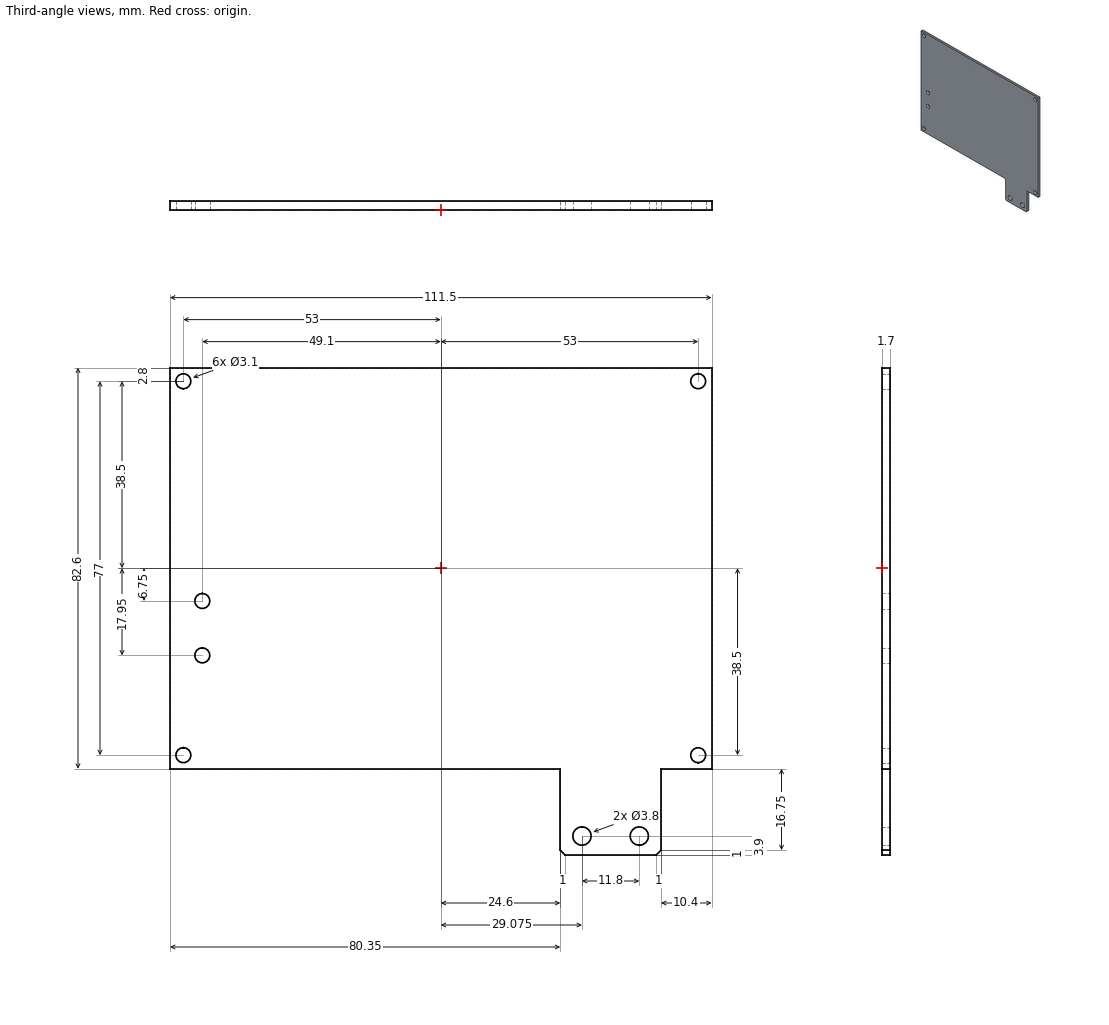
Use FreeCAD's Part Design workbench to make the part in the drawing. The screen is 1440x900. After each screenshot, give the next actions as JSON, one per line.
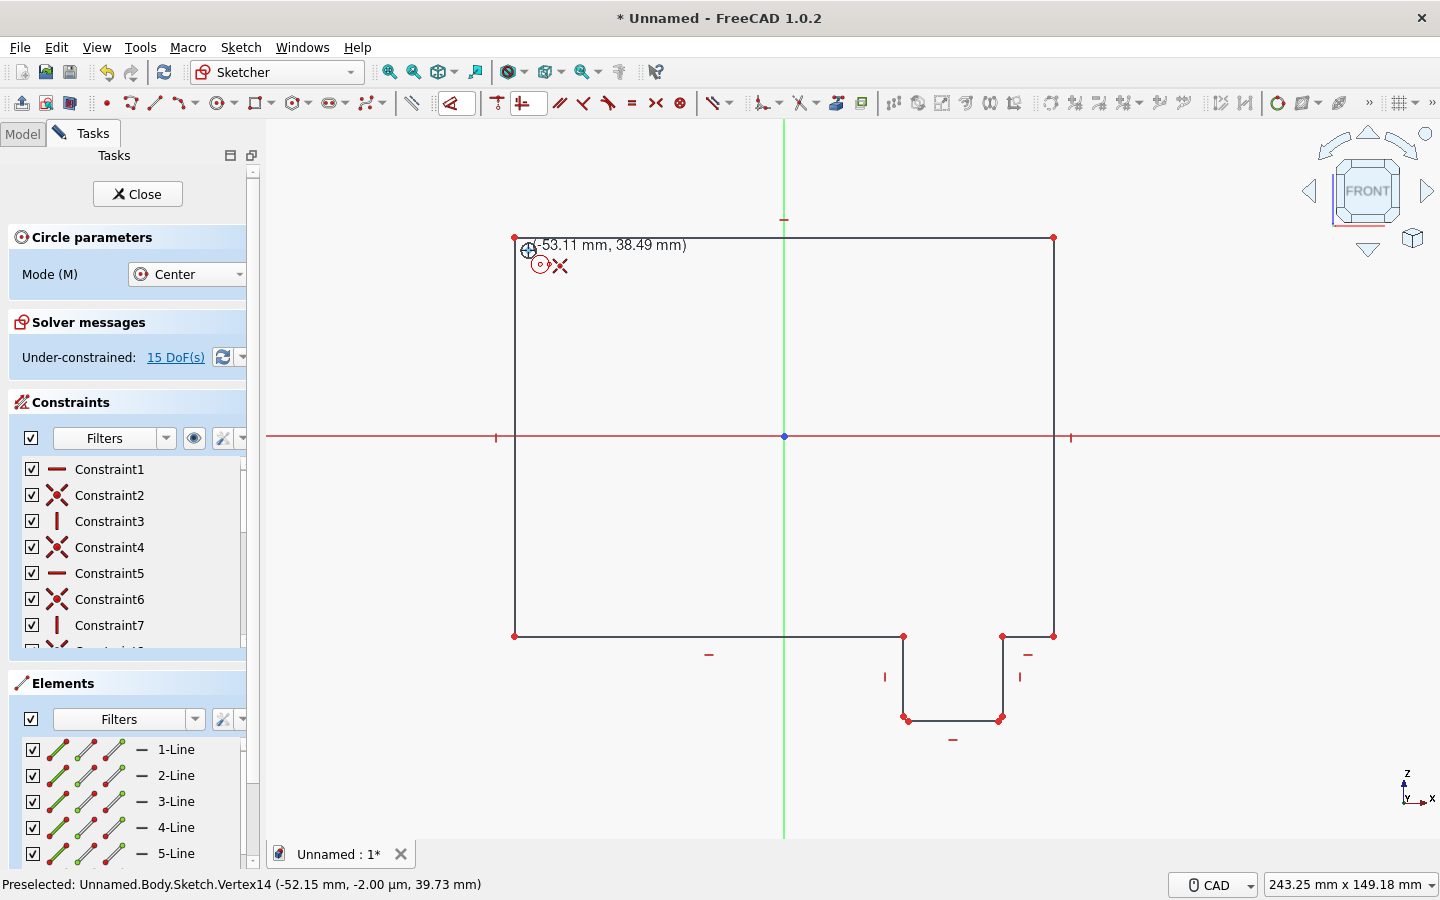
{"action": "scroll", "coordinate": [547, 469], "scroll_direction": "up", "scroll_amount": 6}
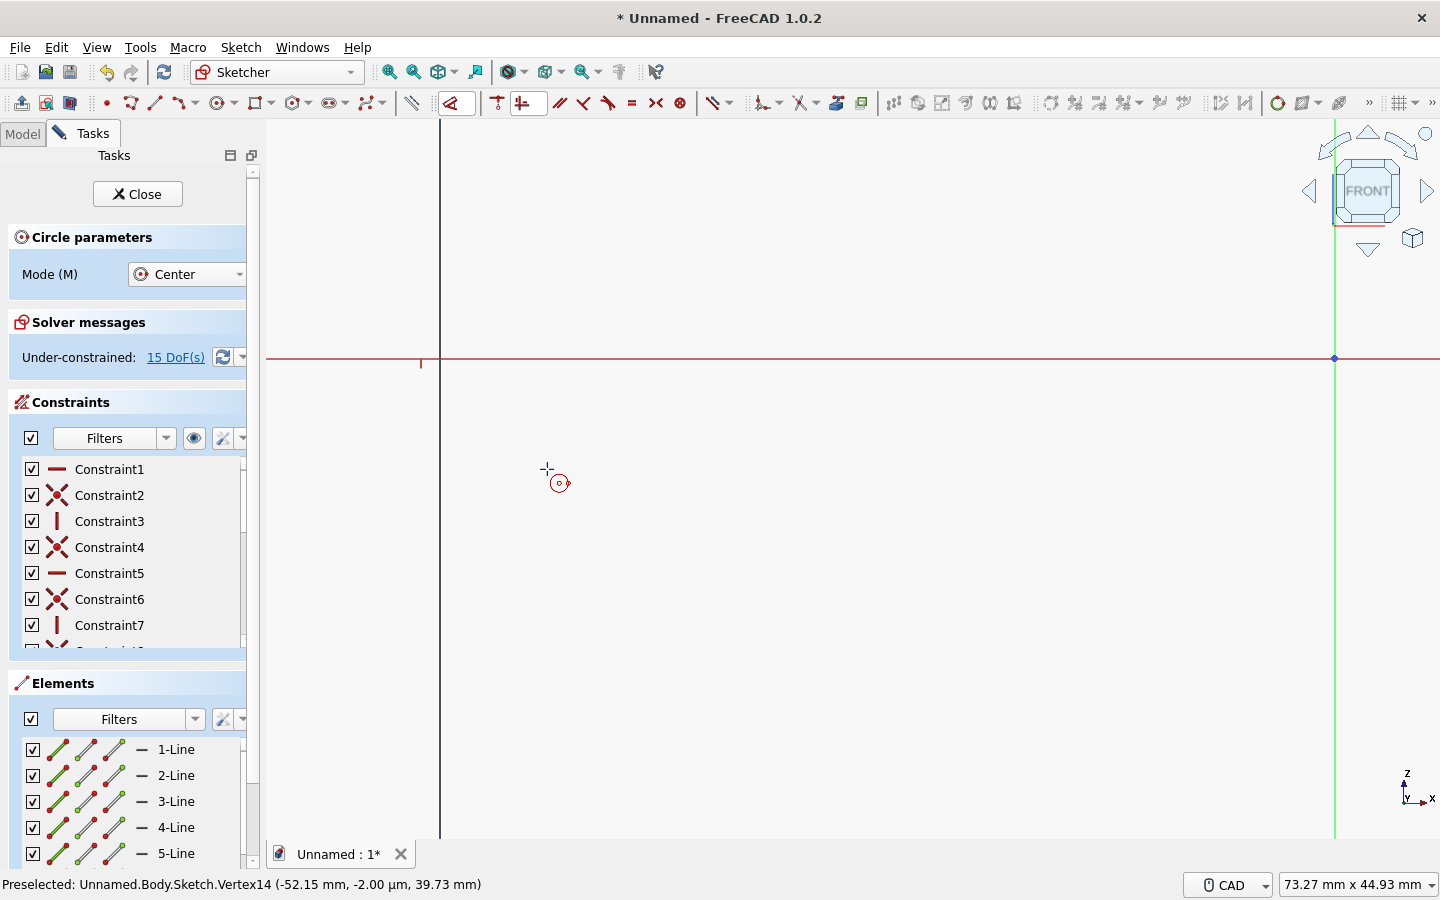
{"action": "left_click", "coordinate": [548, 467]}
{"action": "left_click", "coordinate": [566, 450]}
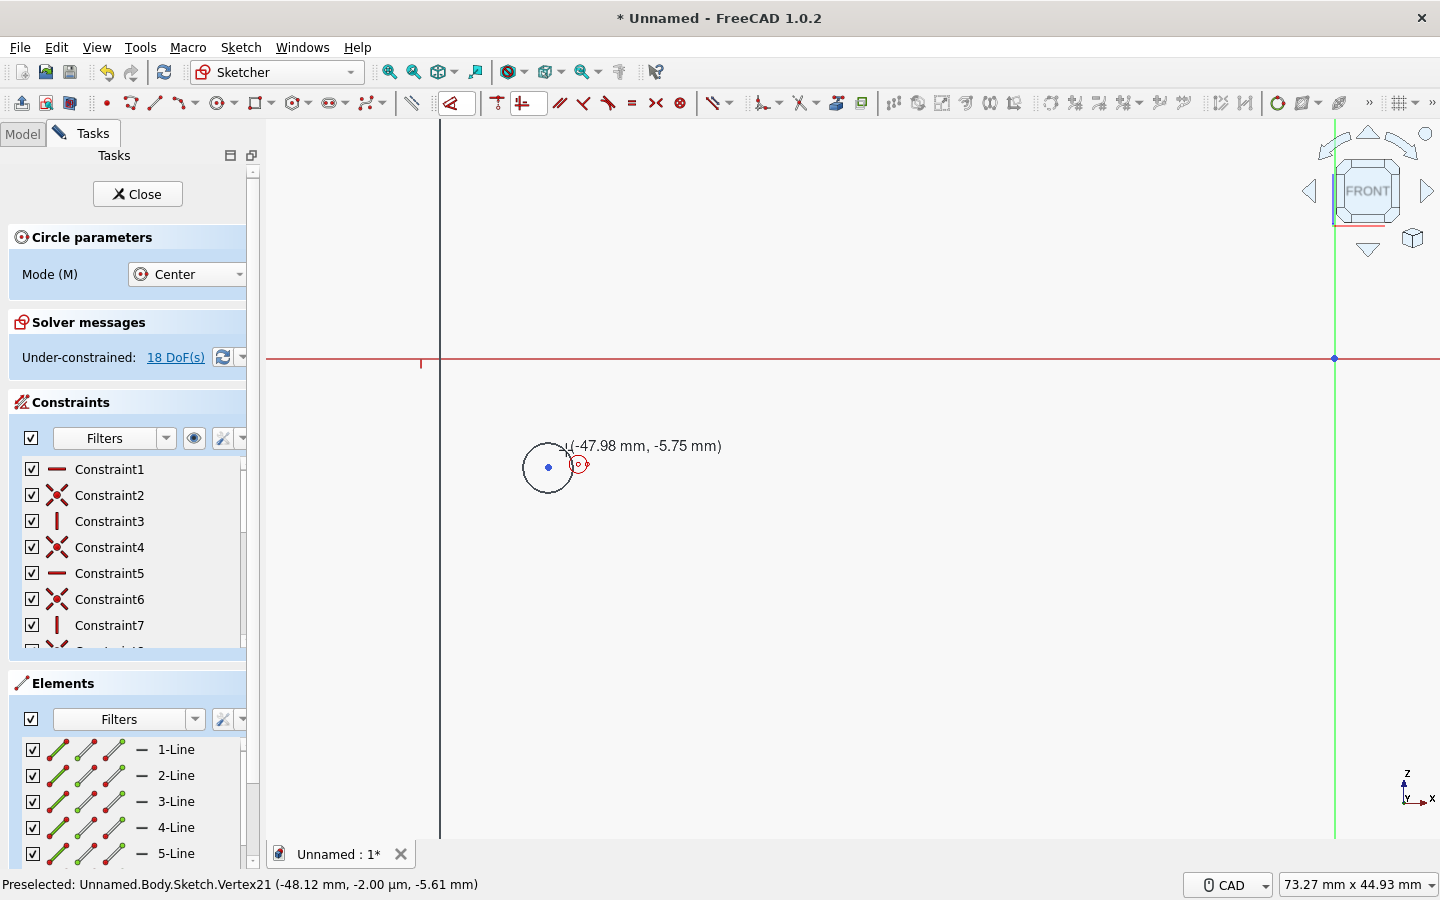
{"action": "scroll", "coordinate": [547, 469], "scroll_direction": "down", "scroll_amount": 6}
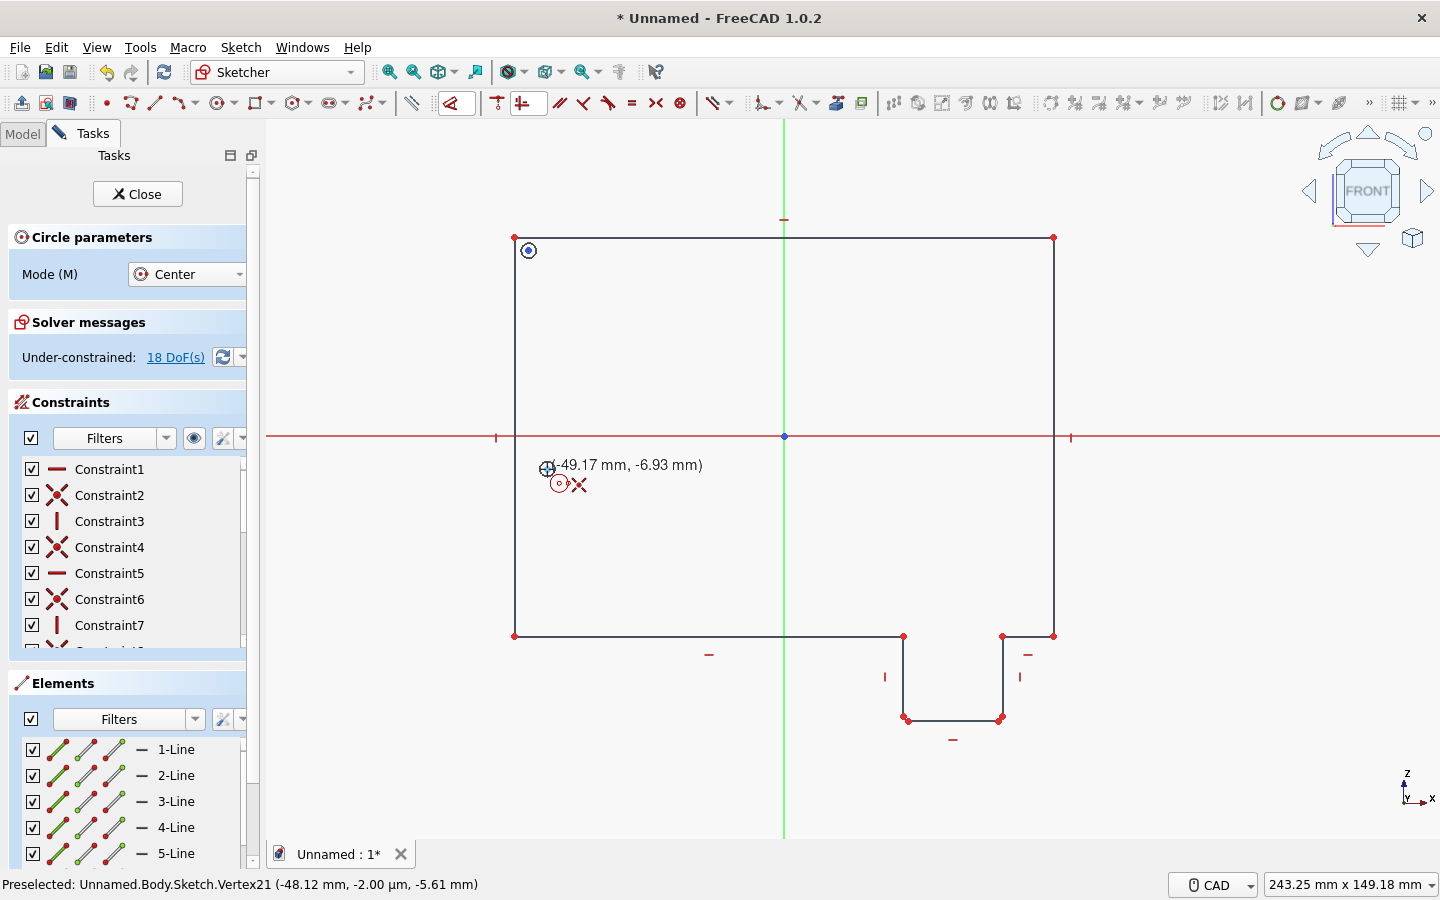
{"action": "scroll", "coordinate": [1040, 250], "scroll_direction": "up", "scroll_amount": 6}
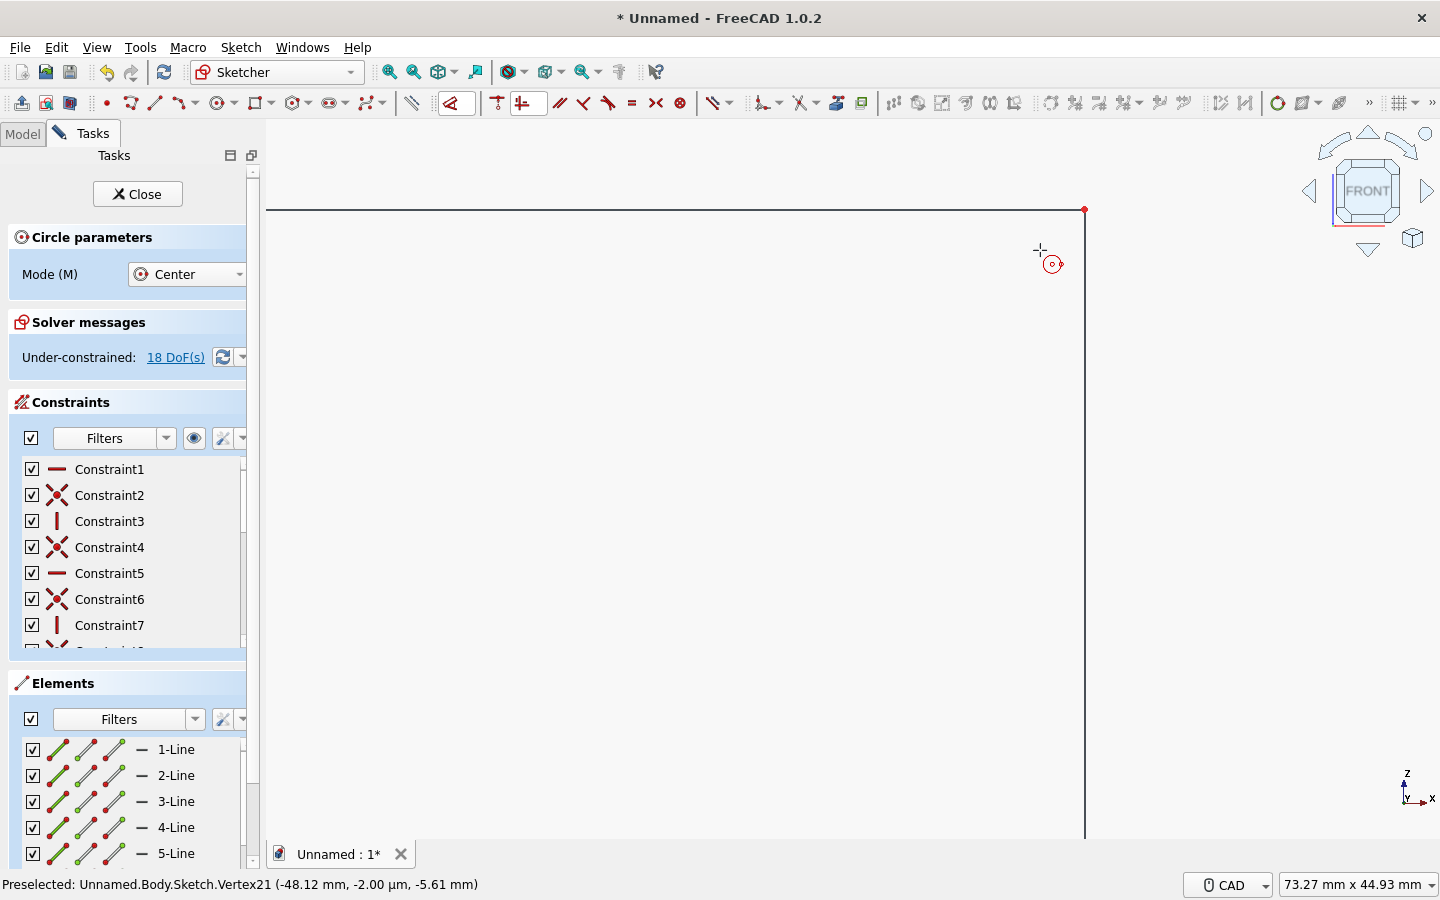
{"action": "left_click", "coordinate": [1039, 251]}
{"action": "left_click", "coordinate": [1057, 233]}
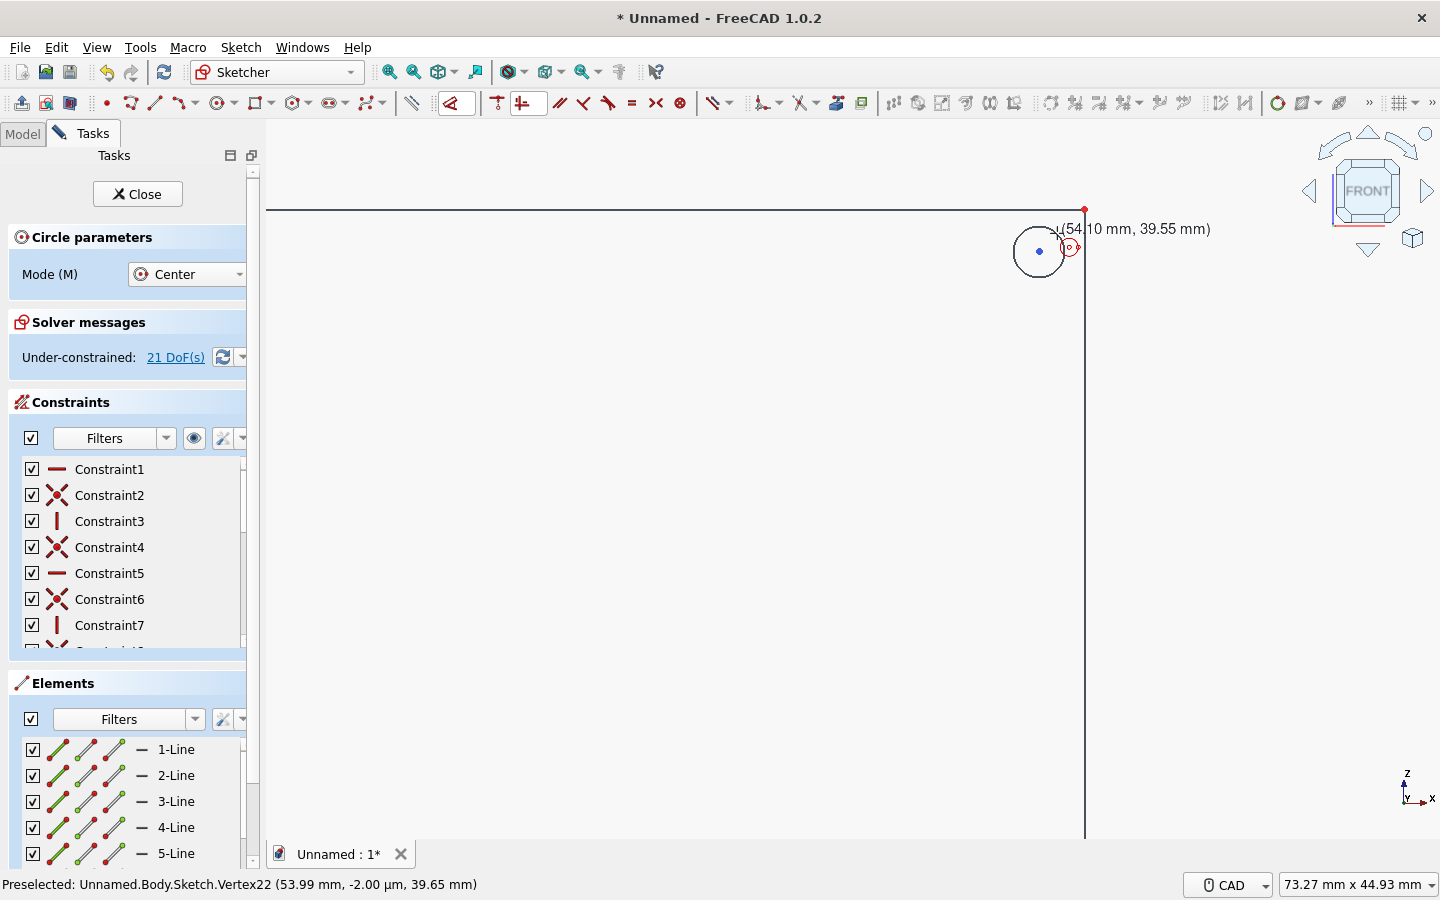
{"action": "scroll", "coordinate": [1041, 250], "scroll_direction": "down", "scroll_amount": 6}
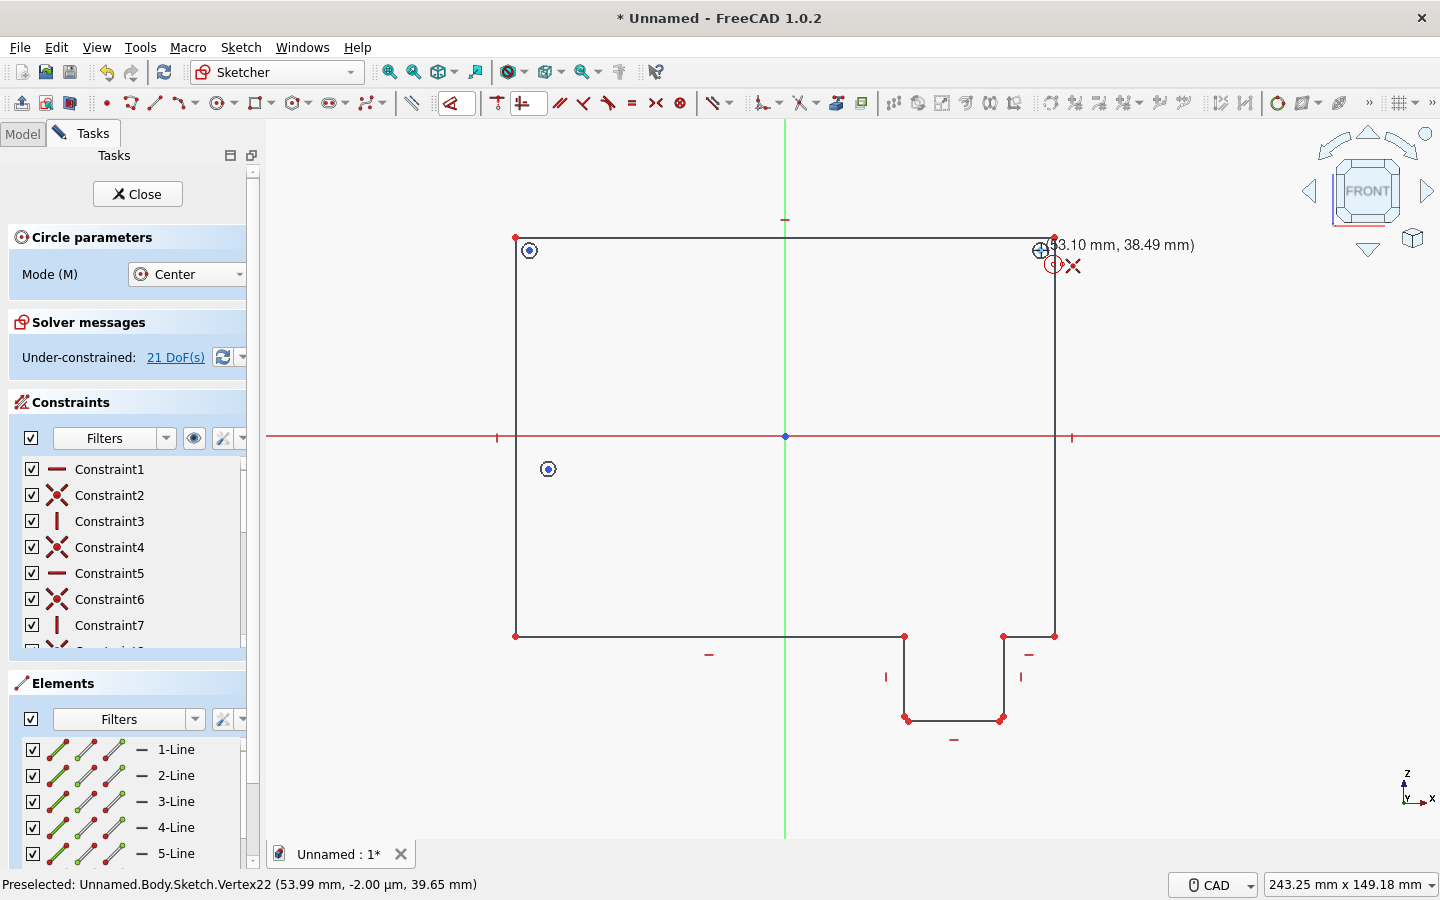
{"action": "scroll", "coordinate": [548, 523], "scroll_direction": "up", "scroll_amount": 6}